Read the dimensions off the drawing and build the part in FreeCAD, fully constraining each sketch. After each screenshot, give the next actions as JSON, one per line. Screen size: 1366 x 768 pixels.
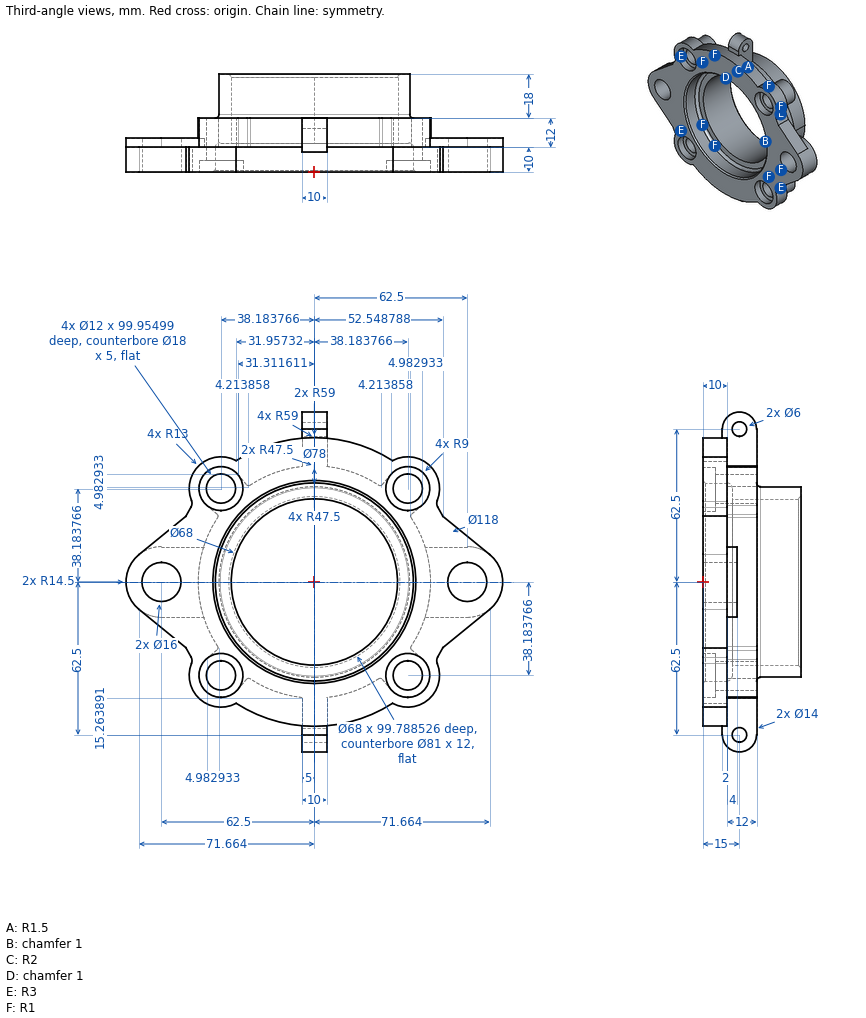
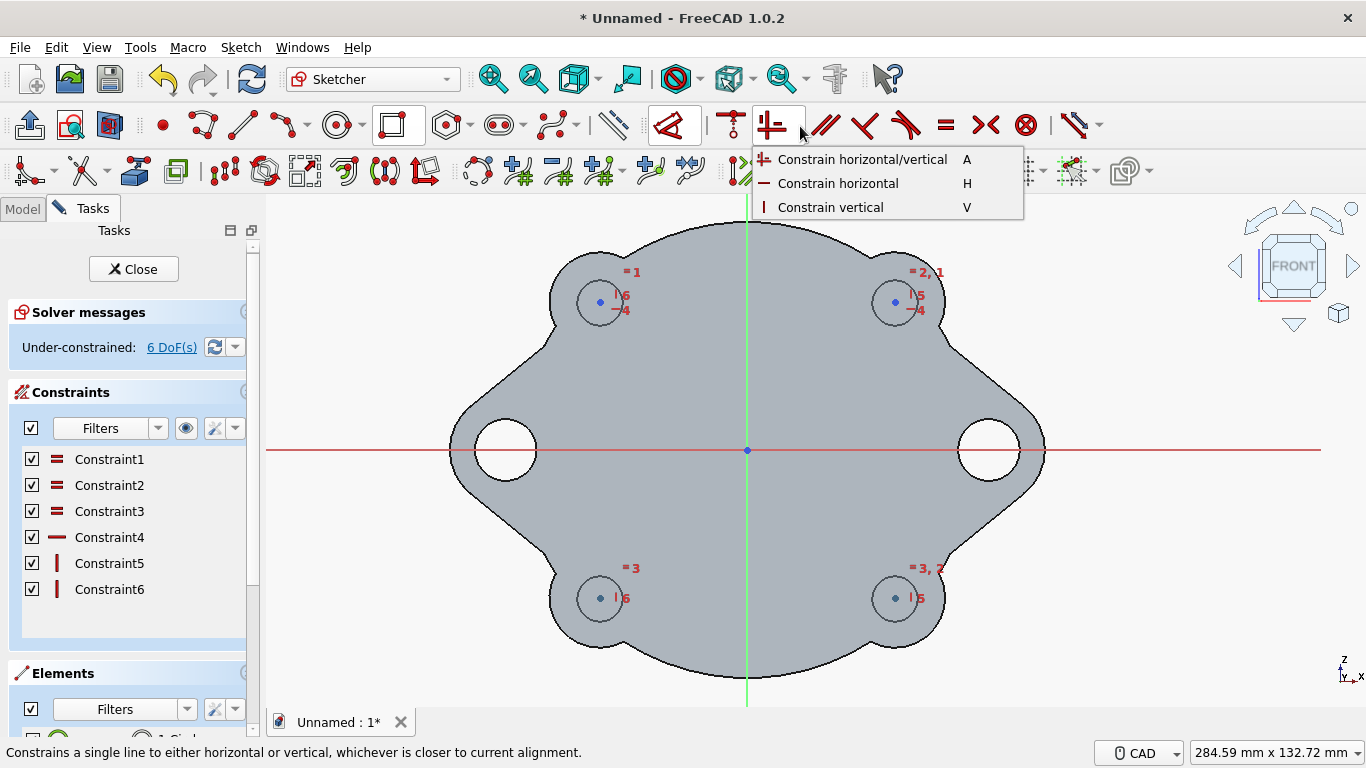
{"action": "left_click", "coordinate": [888, 183]}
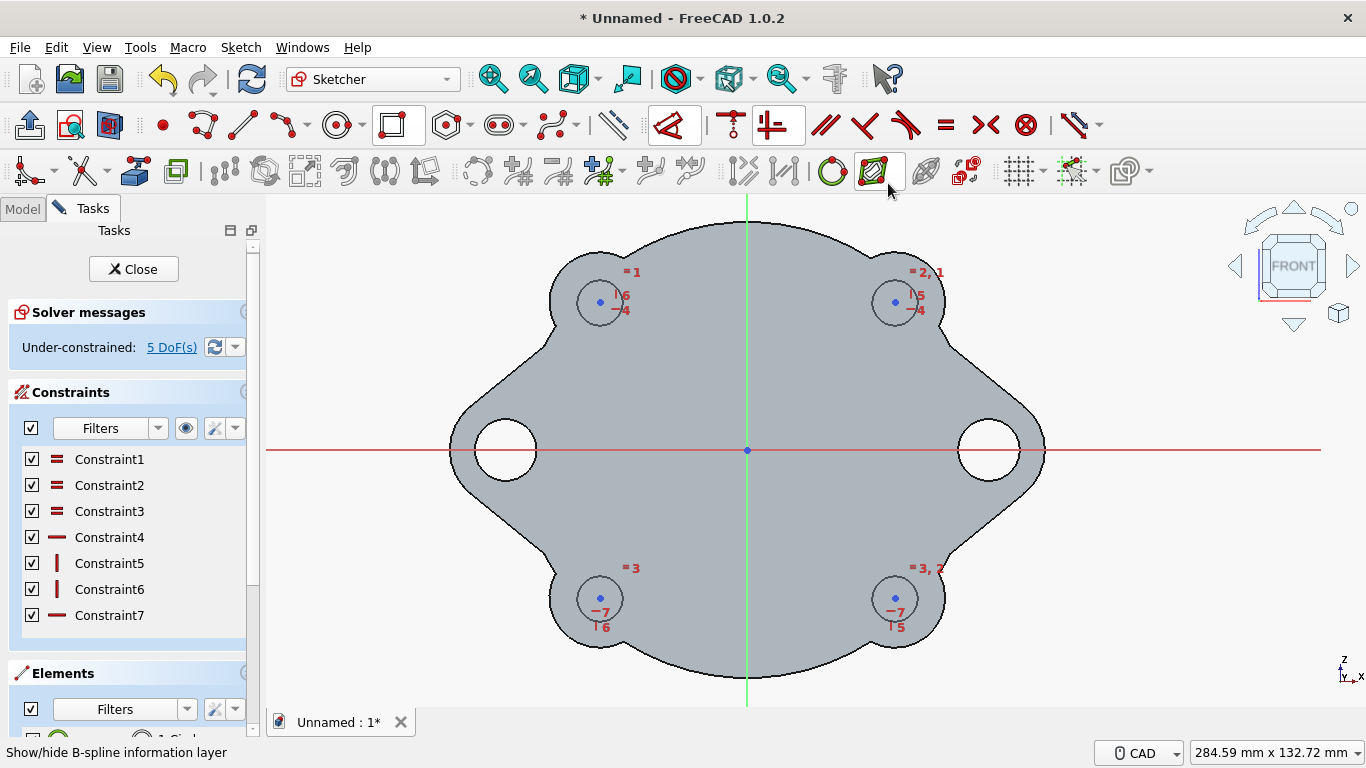
{"action": "left_click", "coordinate": [584, 287]}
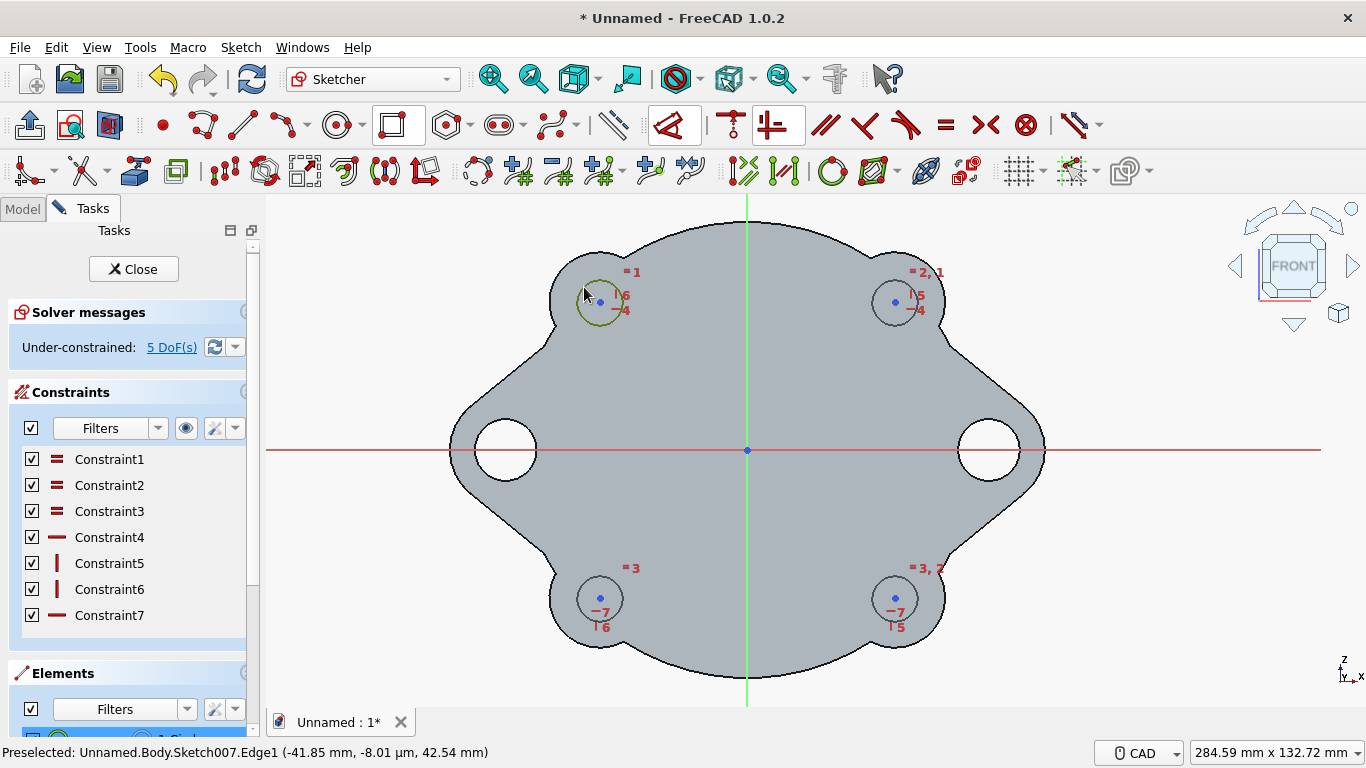
{"action": "left_click", "coordinate": [696, 126]}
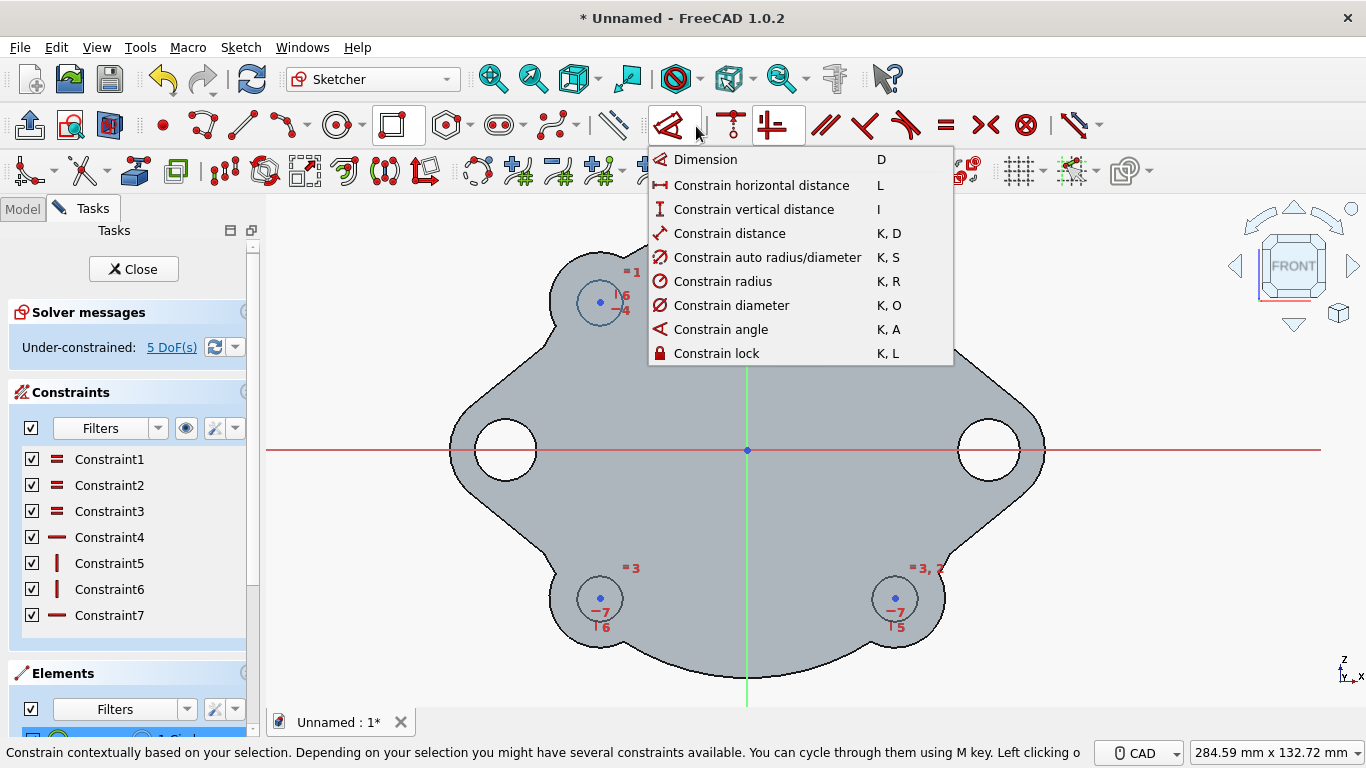
{"action": "left_click", "coordinate": [801, 305]}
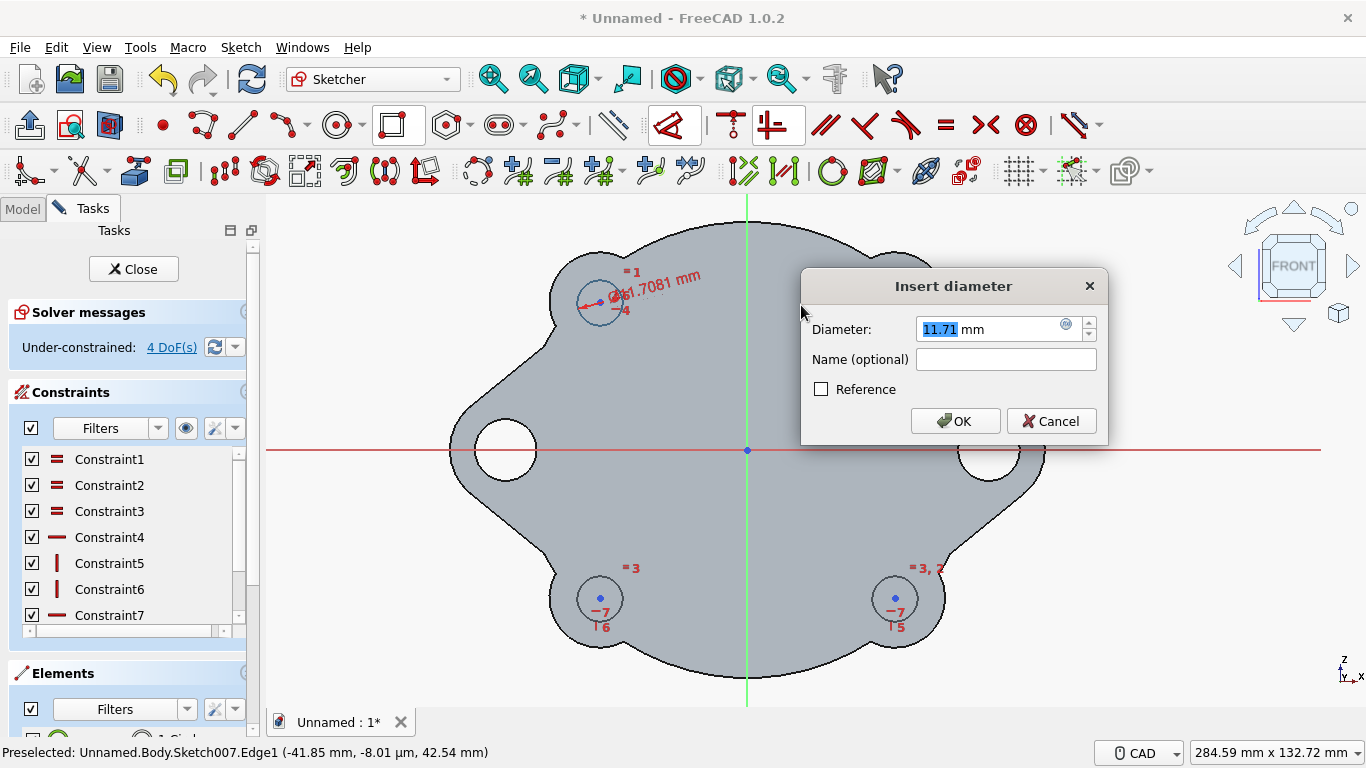
{"action": "type", "text": "12"}
{"action": "key", "text": "Return"}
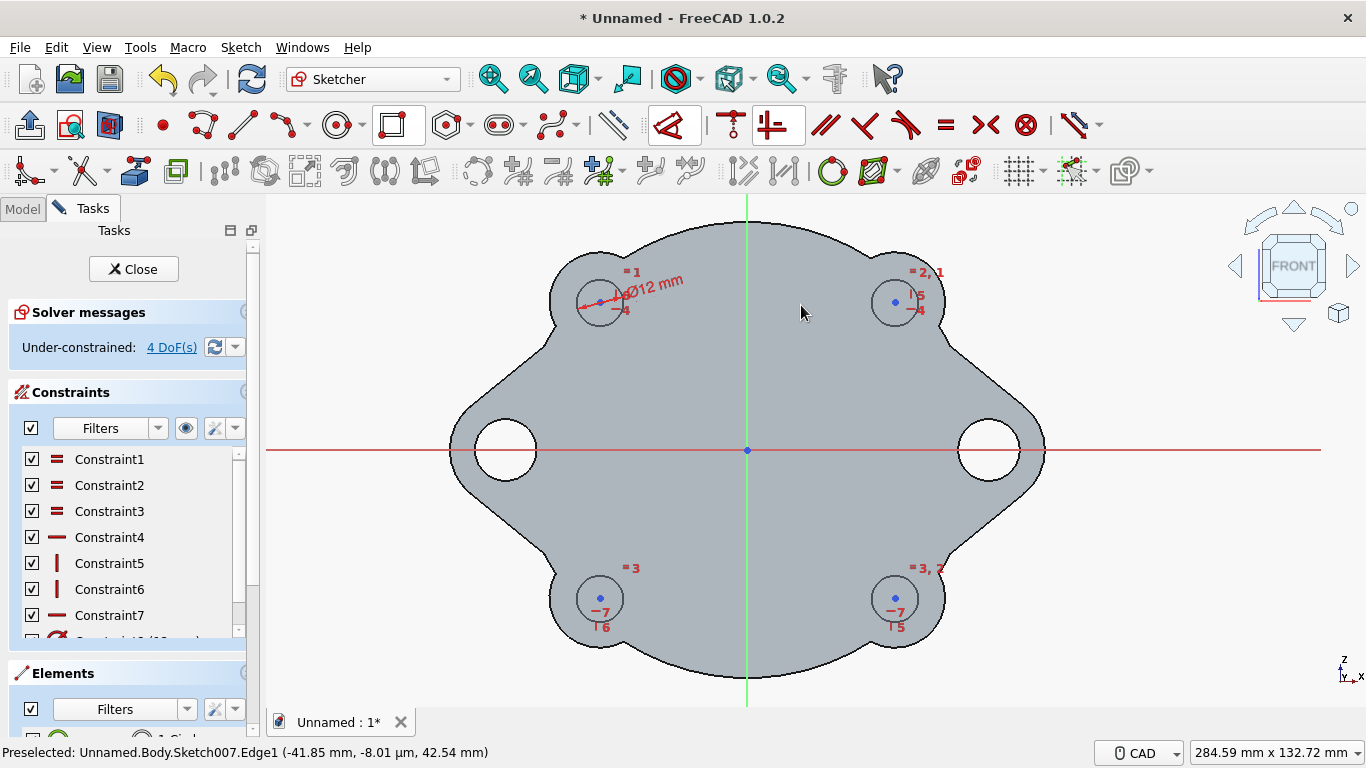
{"action": "left_click", "coordinate": [600, 303]}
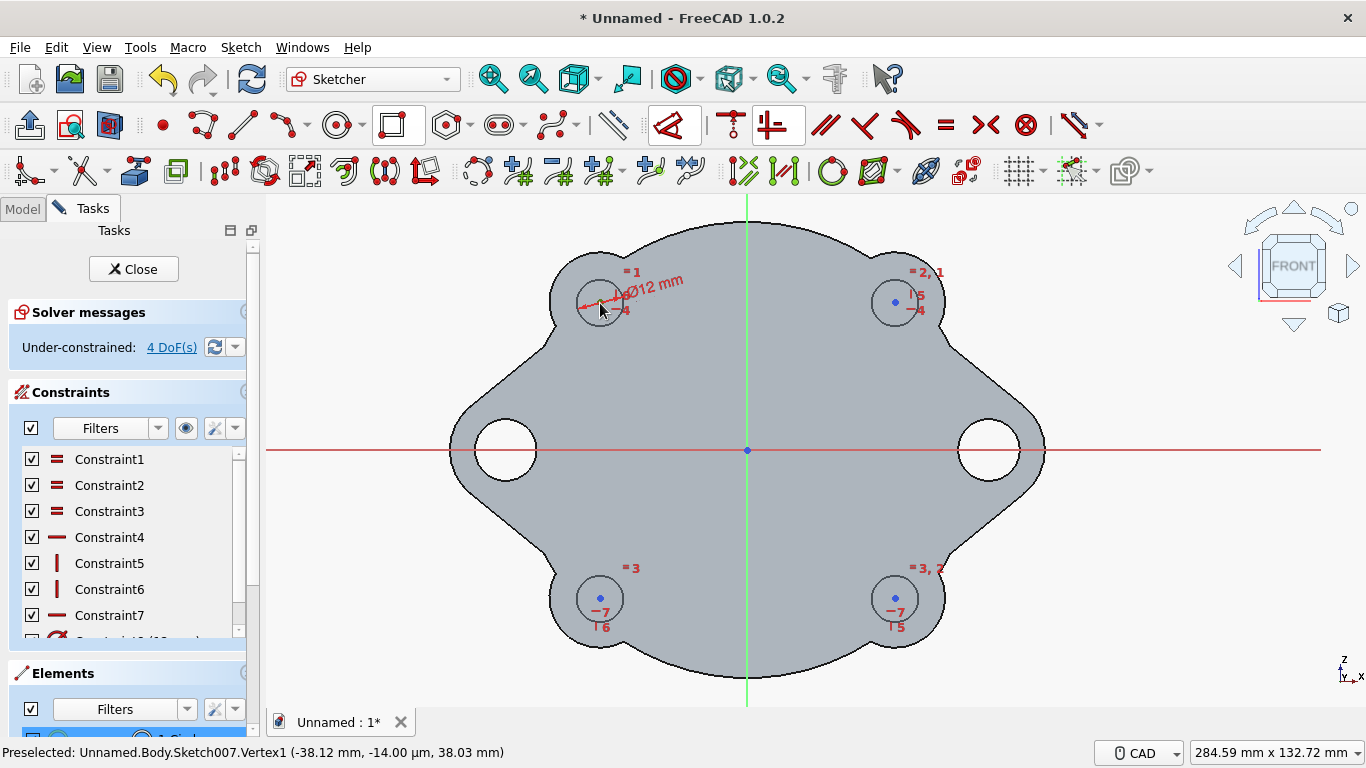
{"action": "left_click", "coordinate": [696, 126]}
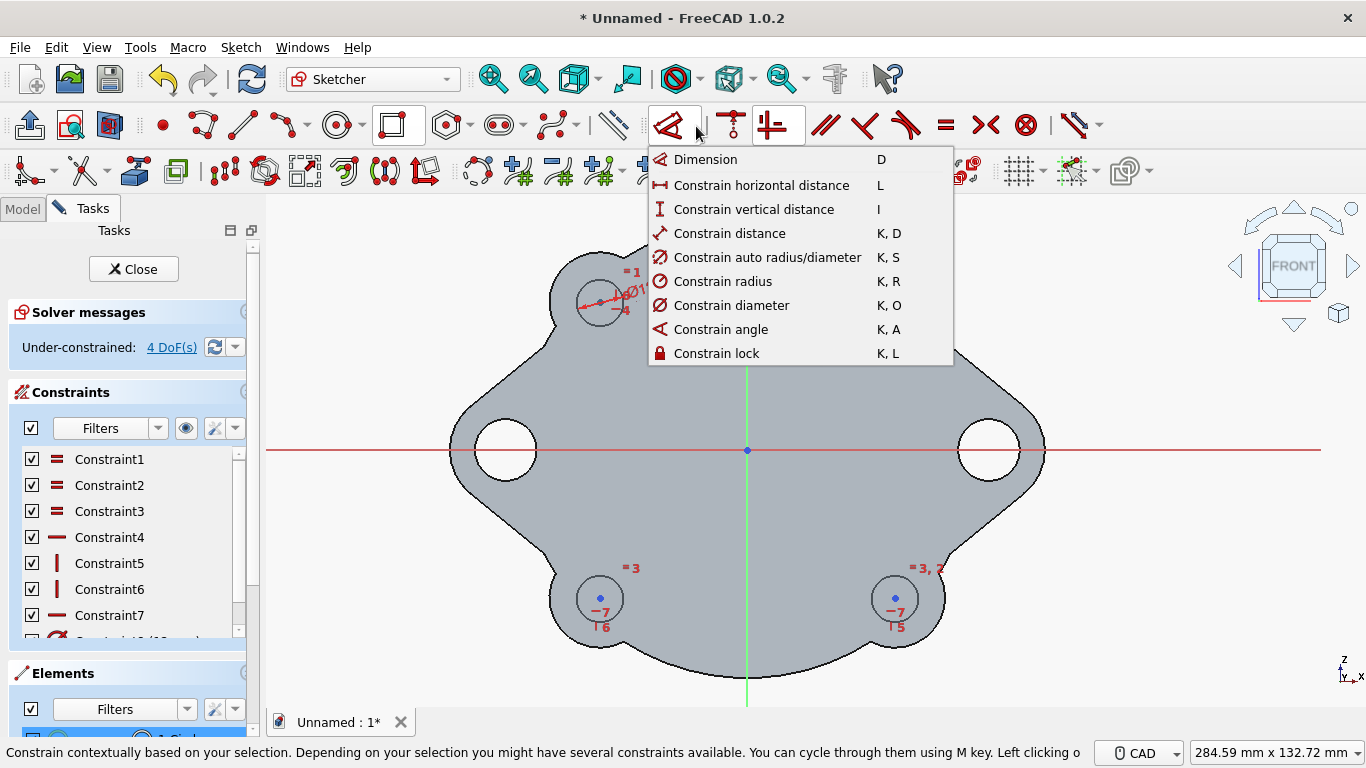
{"action": "left_click", "coordinate": [801, 185]}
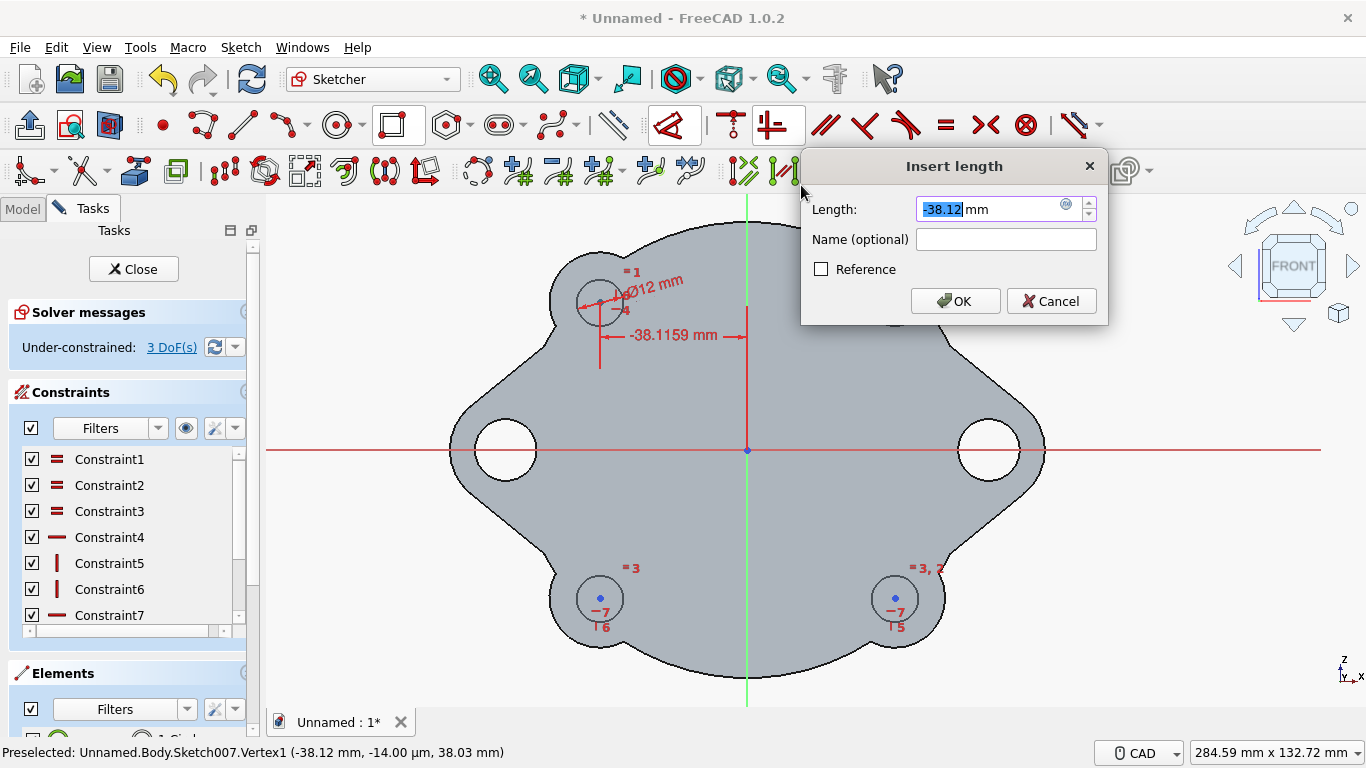
{"action": "type", "text": "-38.183766"}
{"action": "key", "text": "Return"}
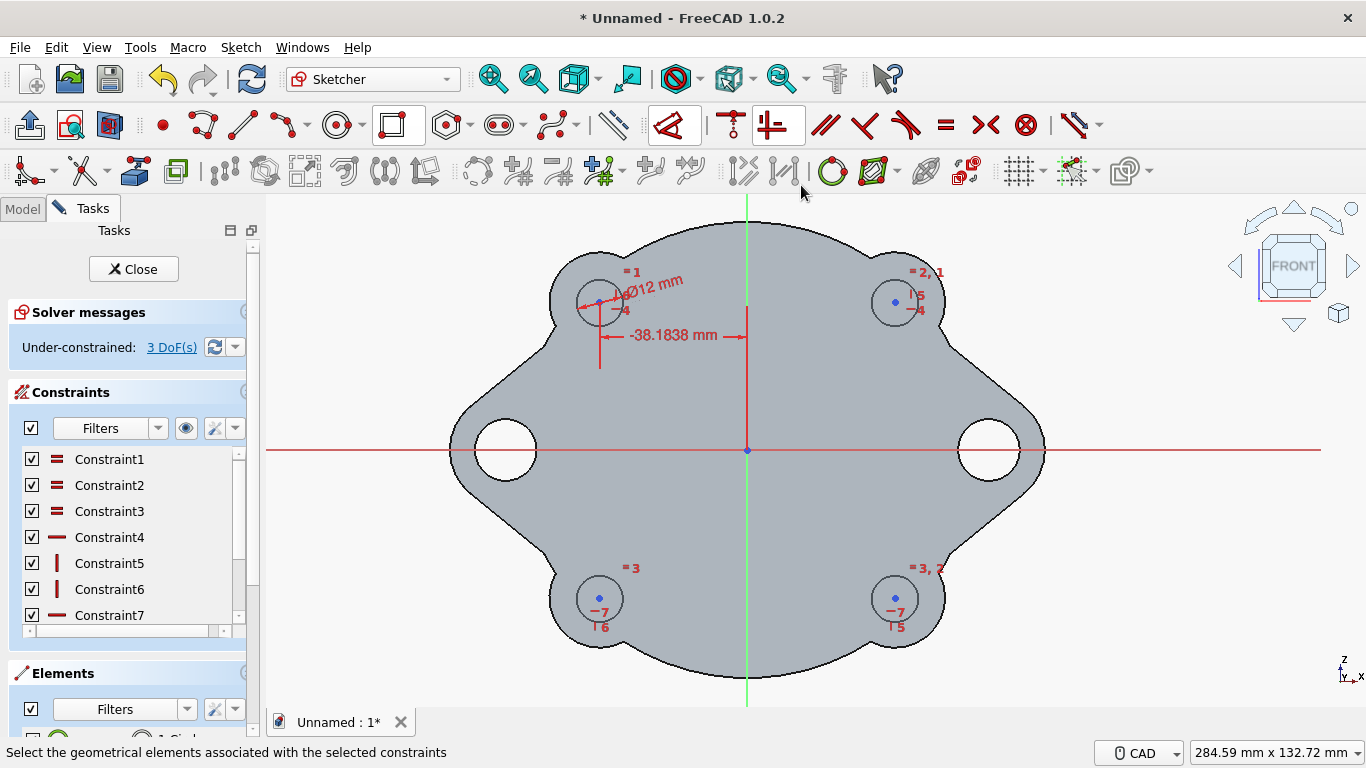
{"action": "left_click", "coordinate": [600, 303]}